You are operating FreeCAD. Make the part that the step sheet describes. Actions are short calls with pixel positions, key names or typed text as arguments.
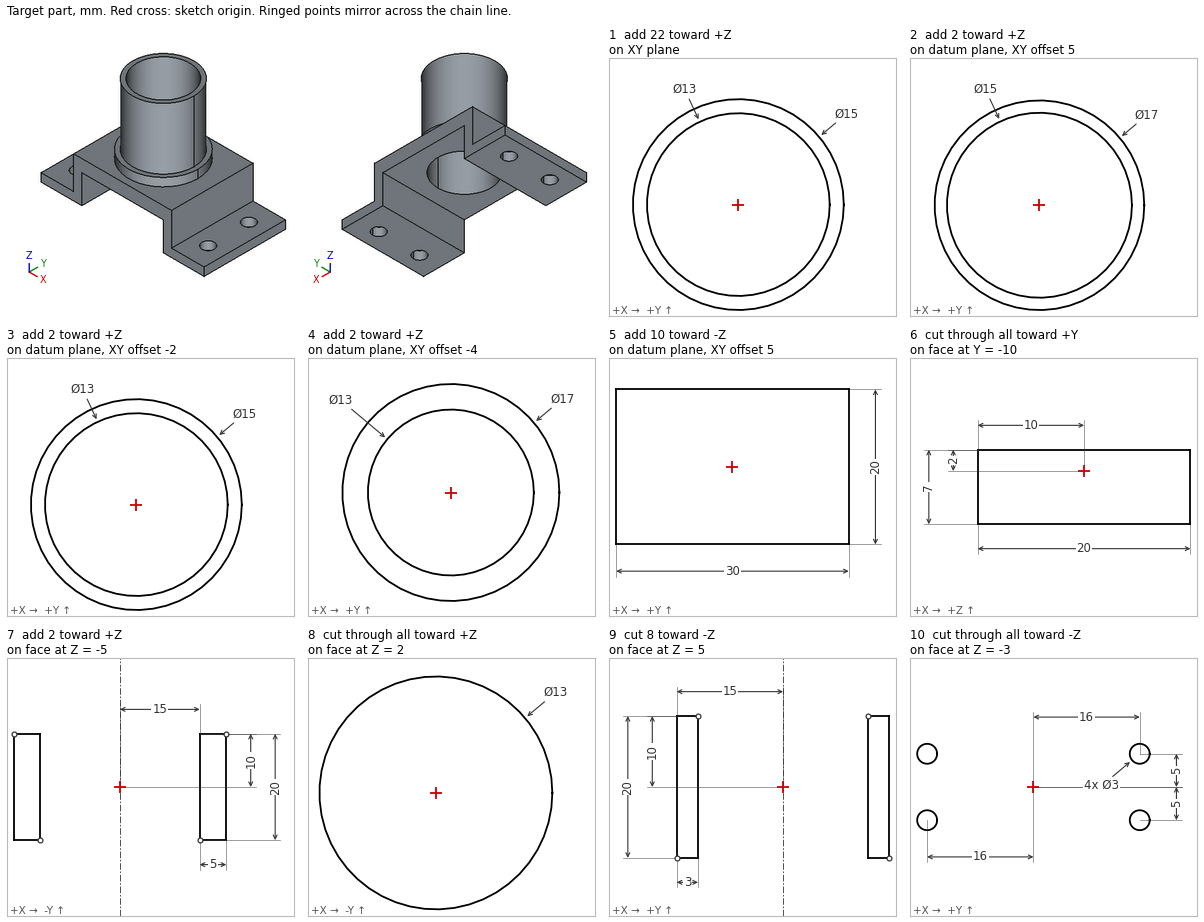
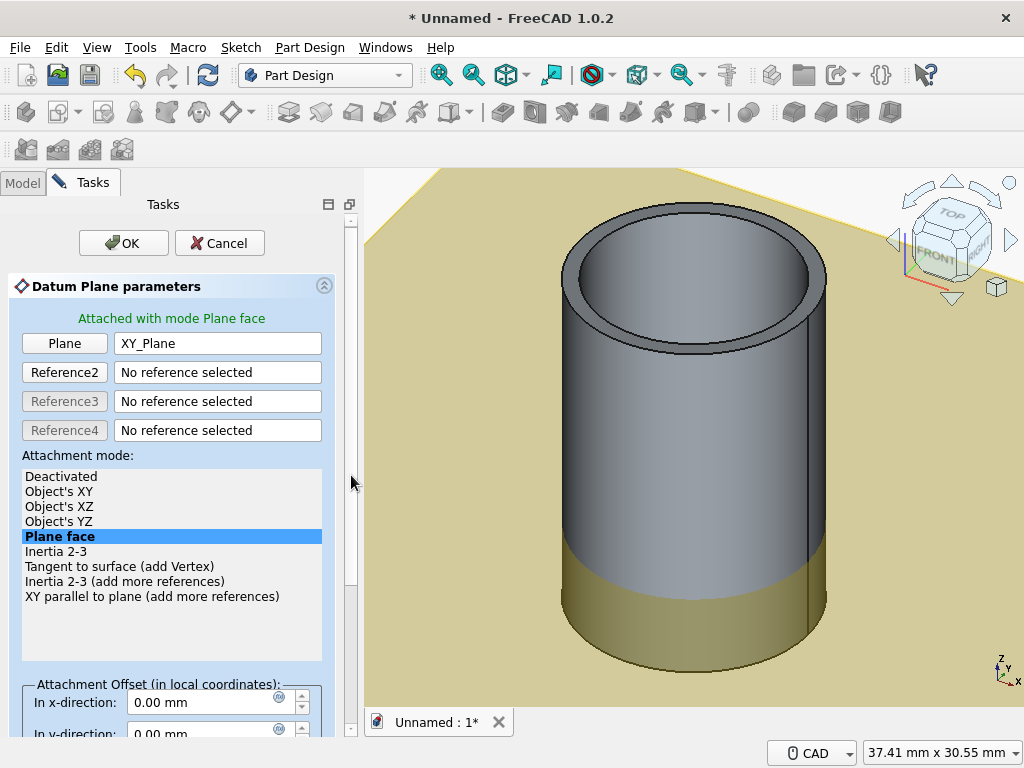
click(124, 243)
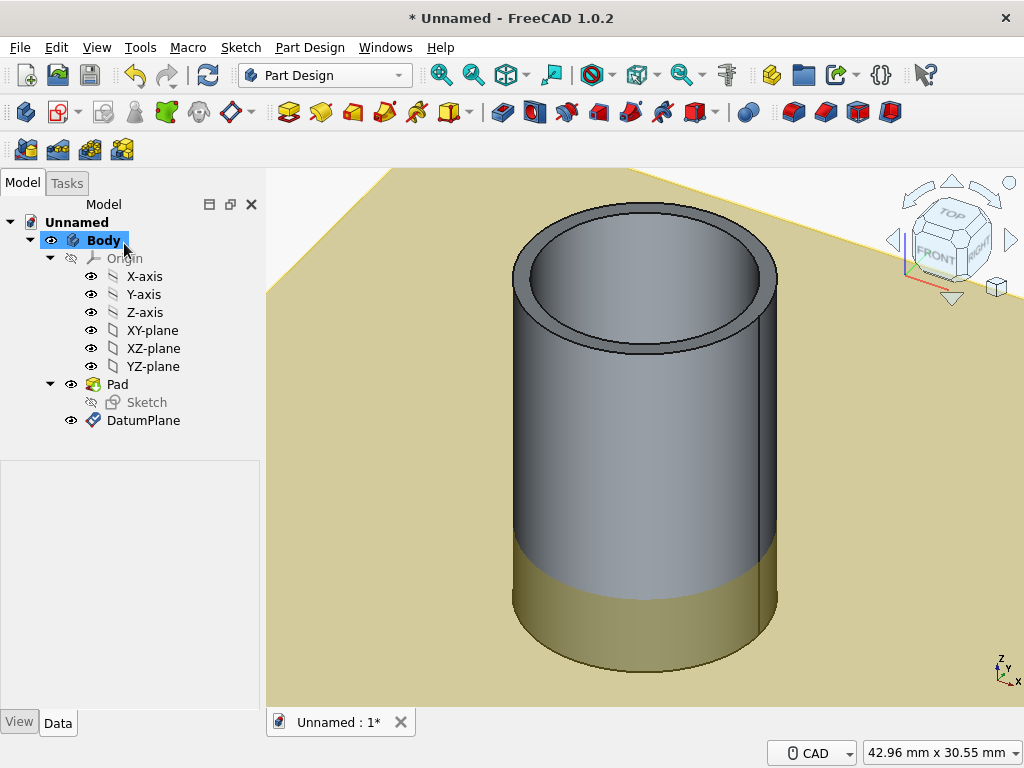
click(116, 420)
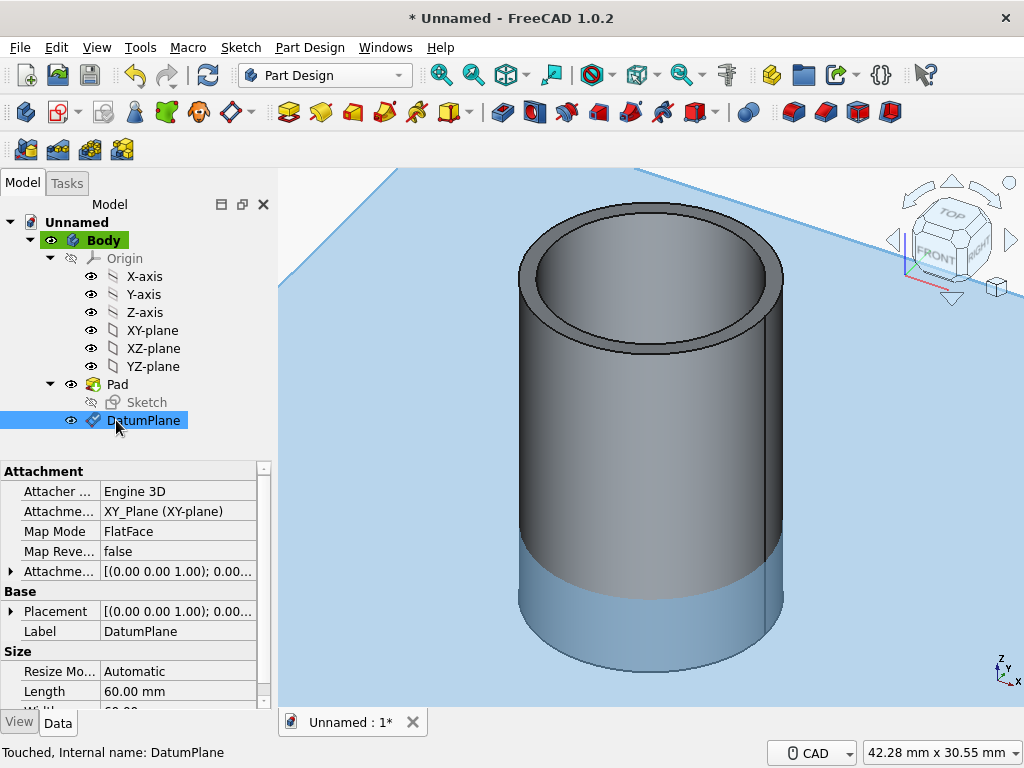
click(58, 112)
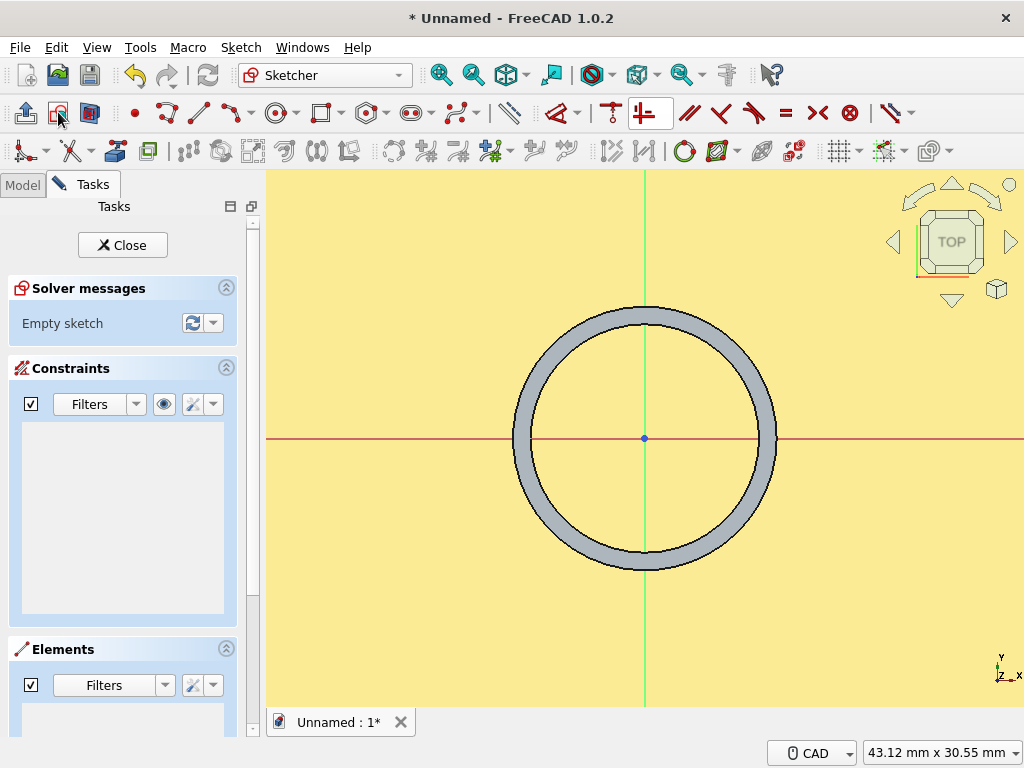
click(90, 114)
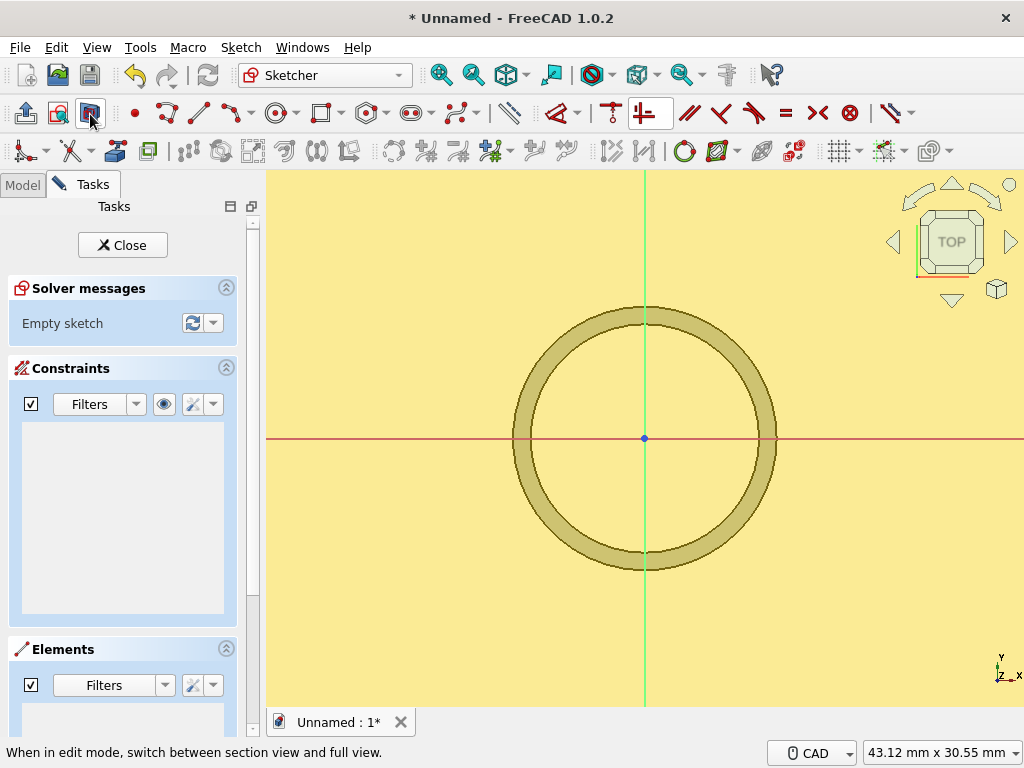
click(276, 114)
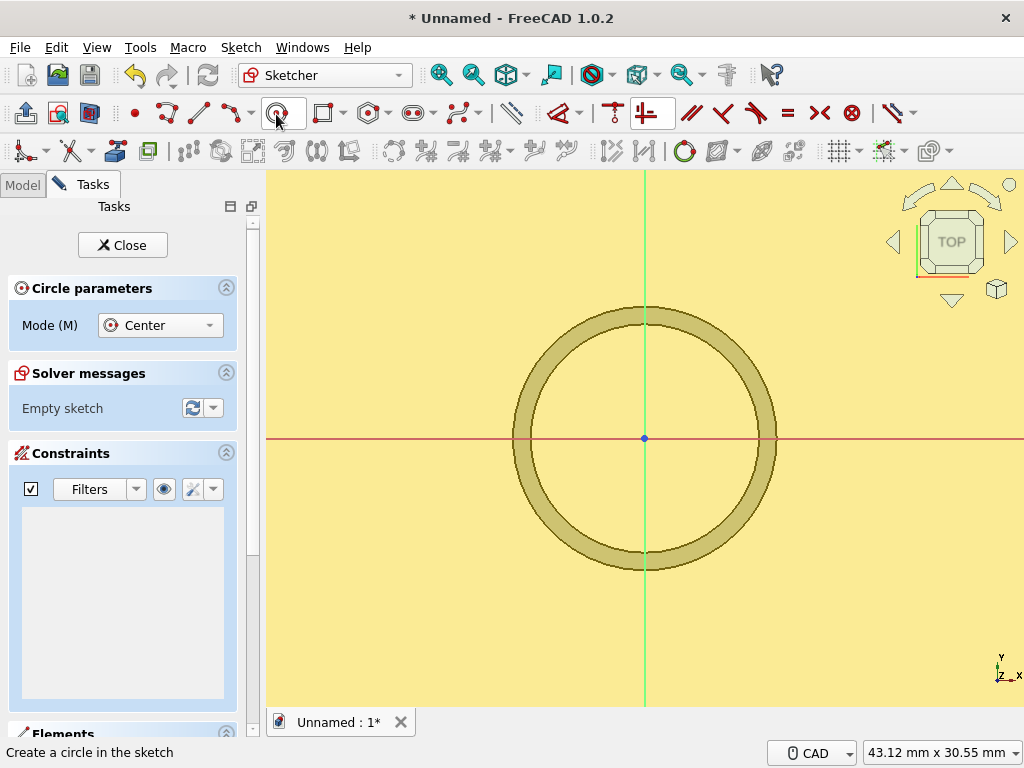
click(645, 438)
click(751, 333)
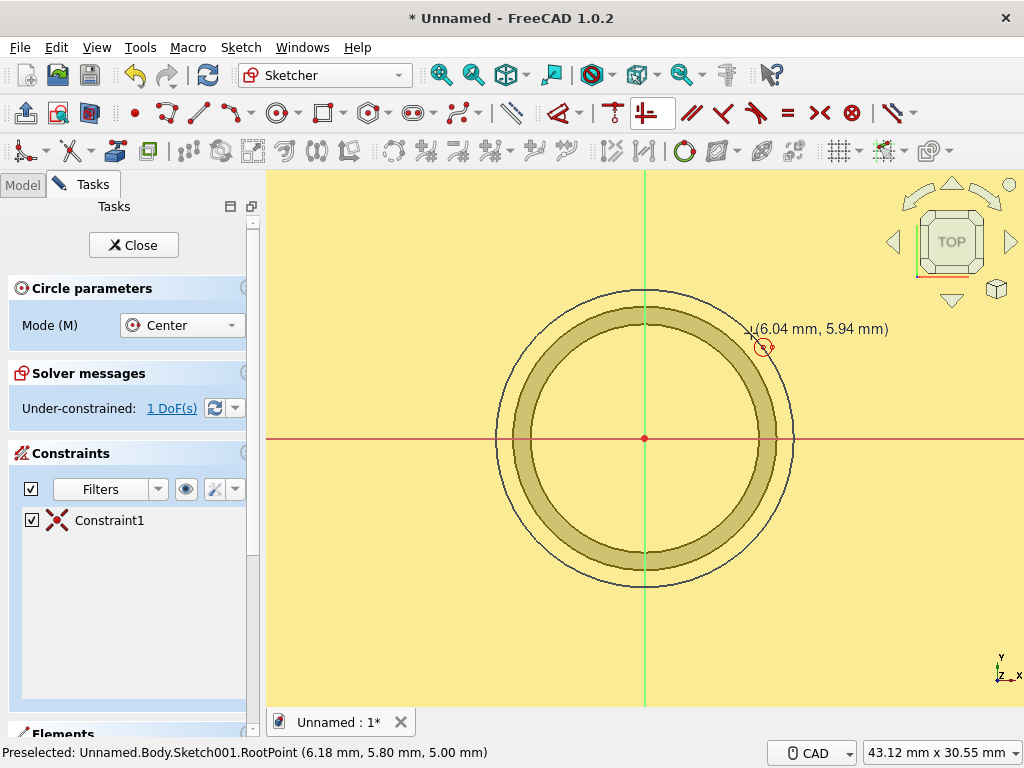
click(645, 438)
click(738, 345)
key(Escape)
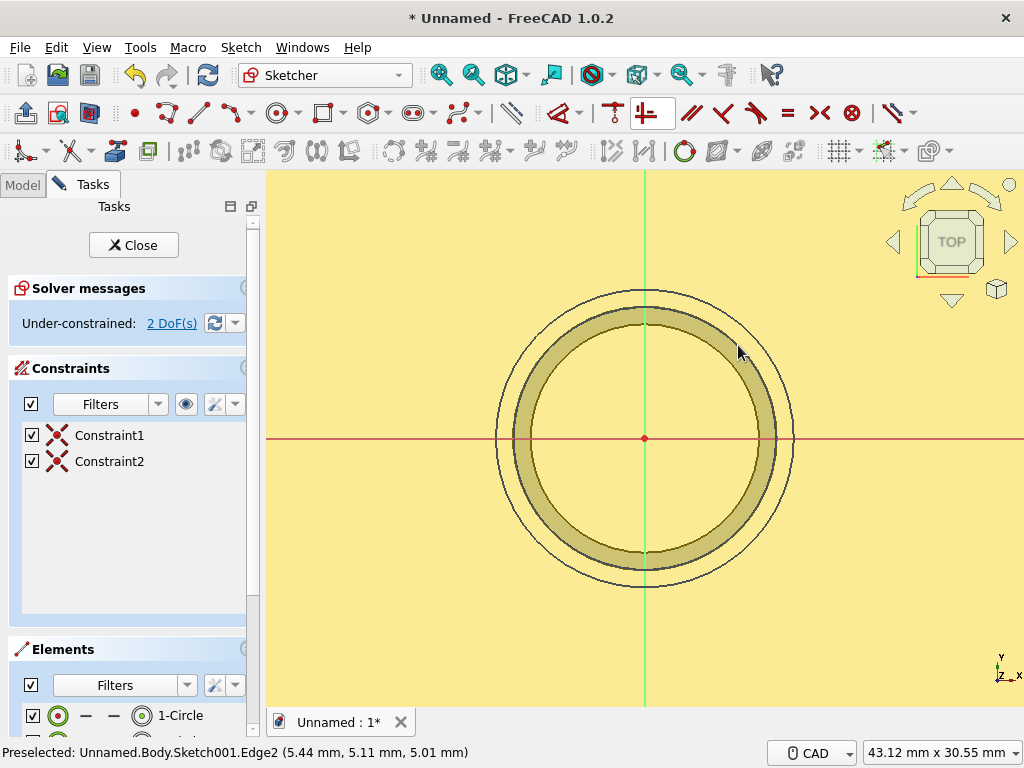
key(d)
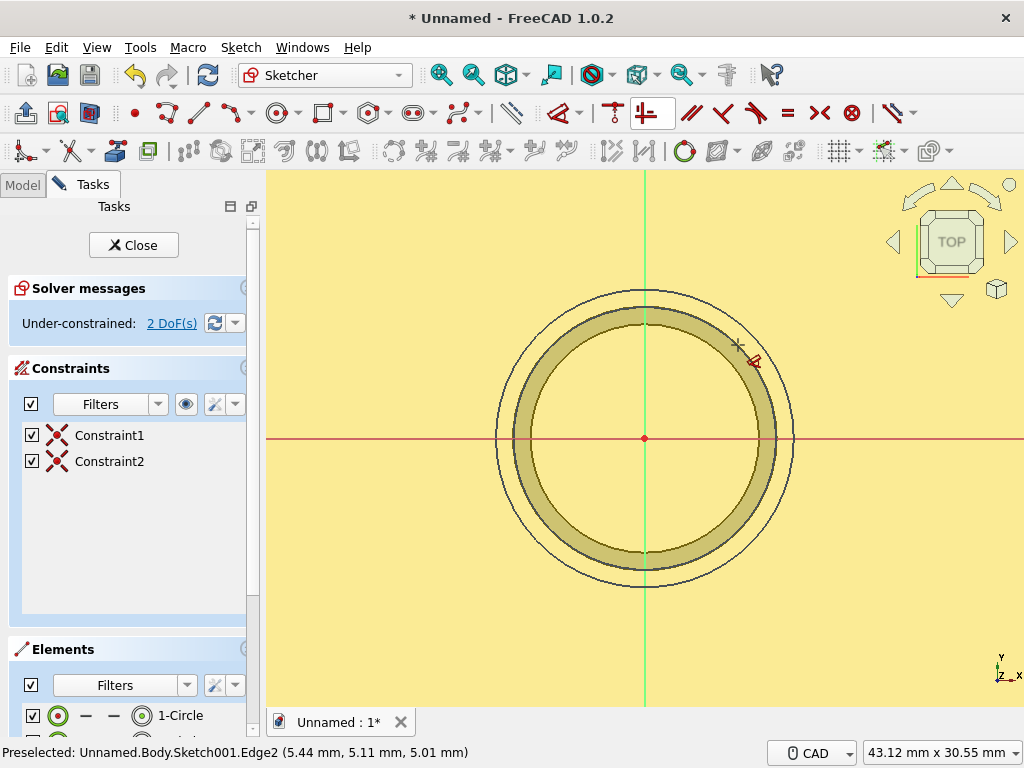
click(750, 333)
click(773, 310)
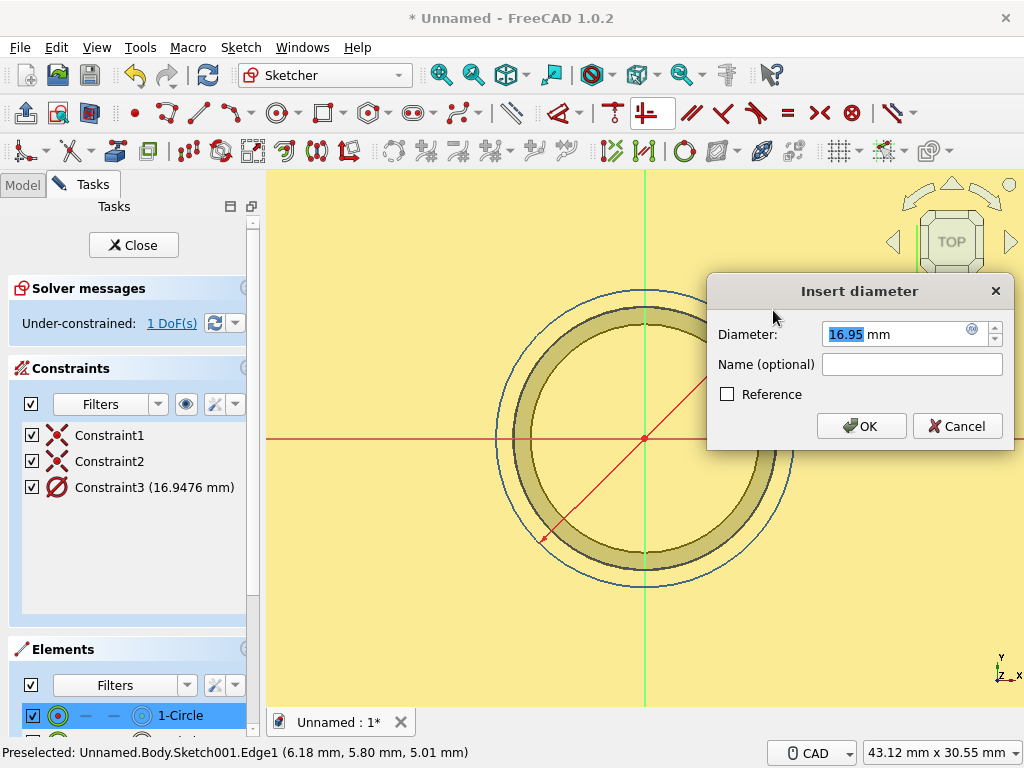
text(17)
key(Return)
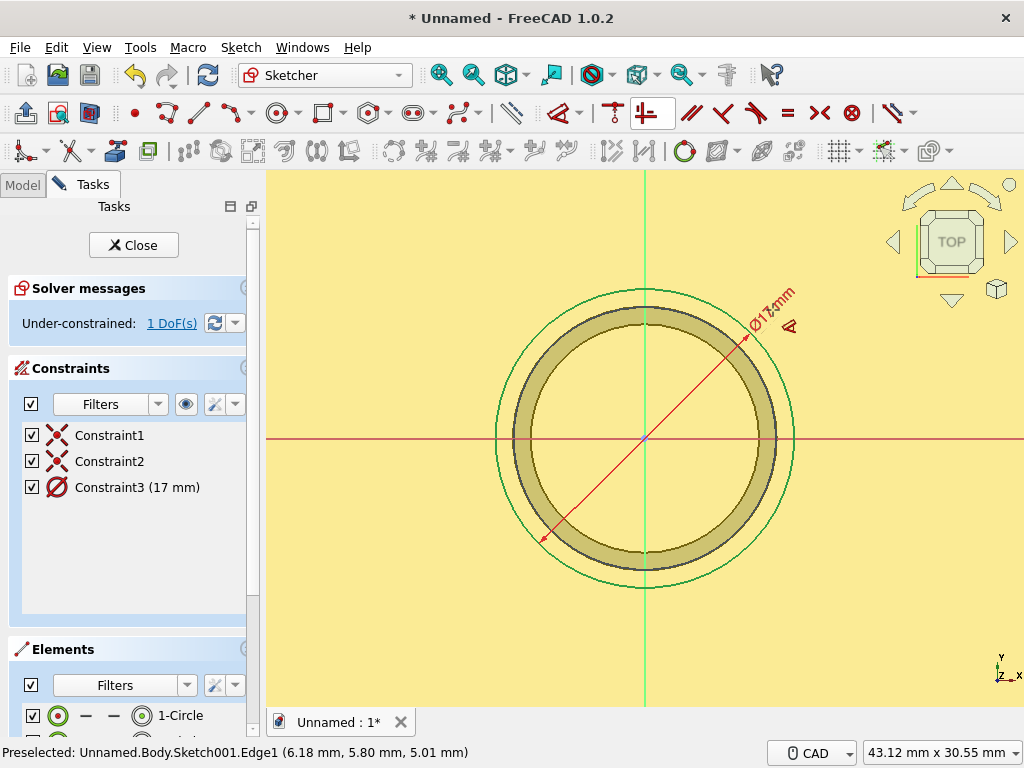
click(737, 345)
click(801, 391)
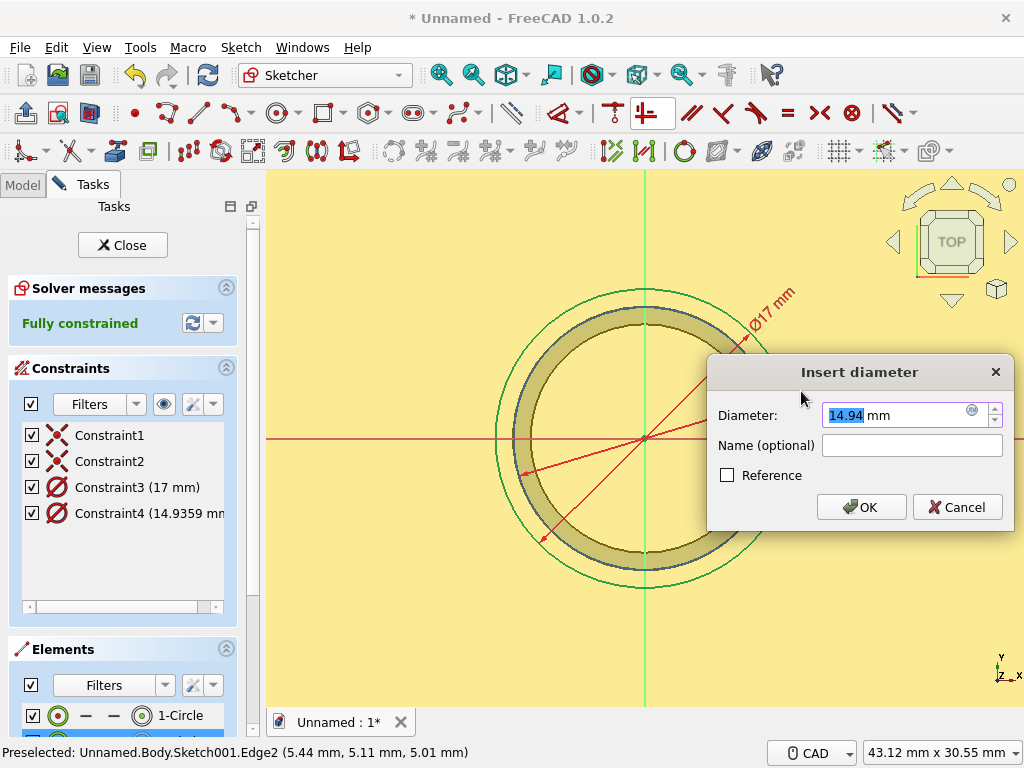
text(15)
key(Return)
key(Escape)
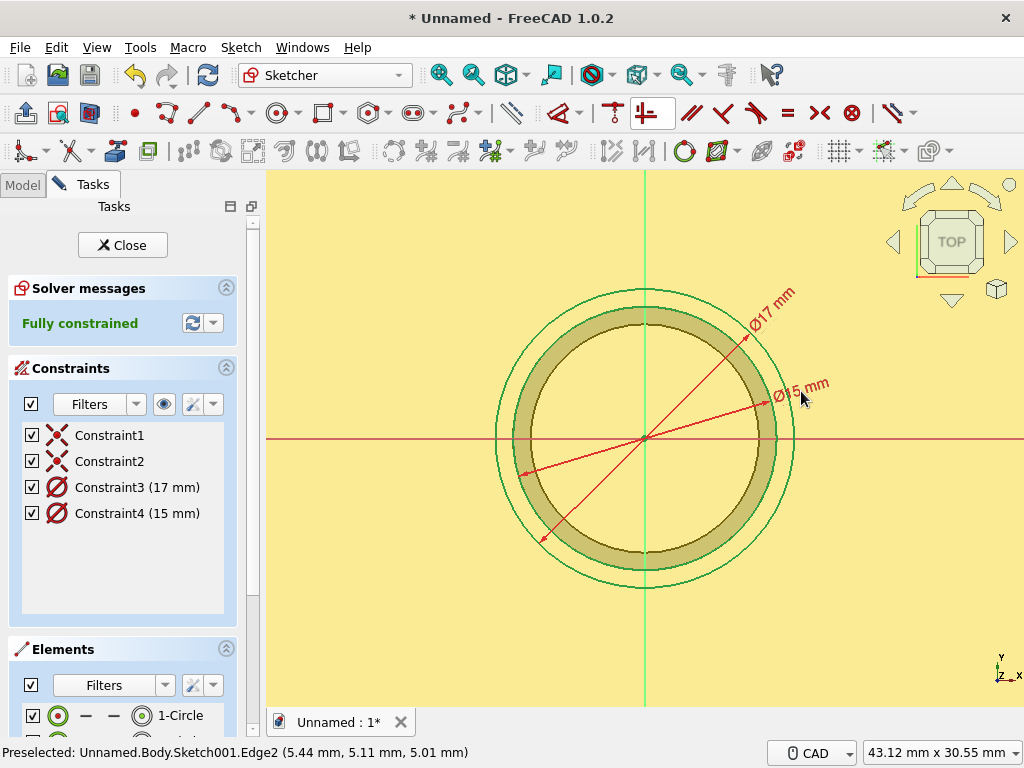
click(123, 245)